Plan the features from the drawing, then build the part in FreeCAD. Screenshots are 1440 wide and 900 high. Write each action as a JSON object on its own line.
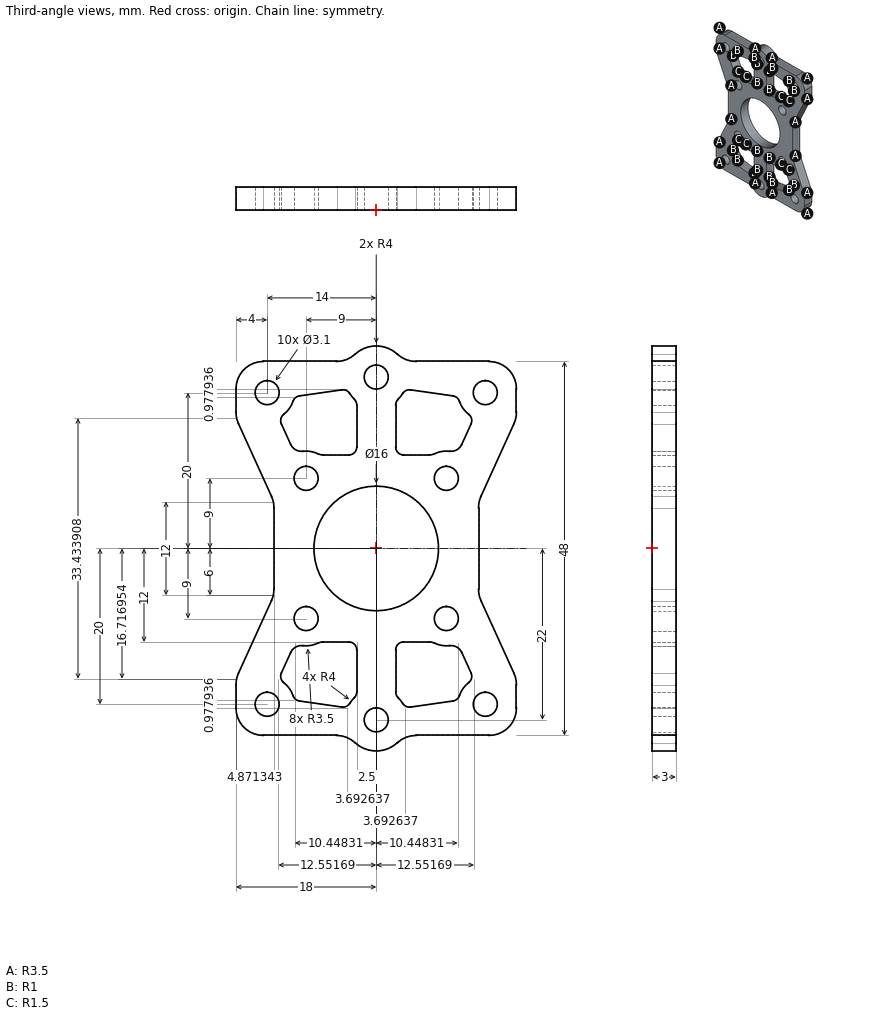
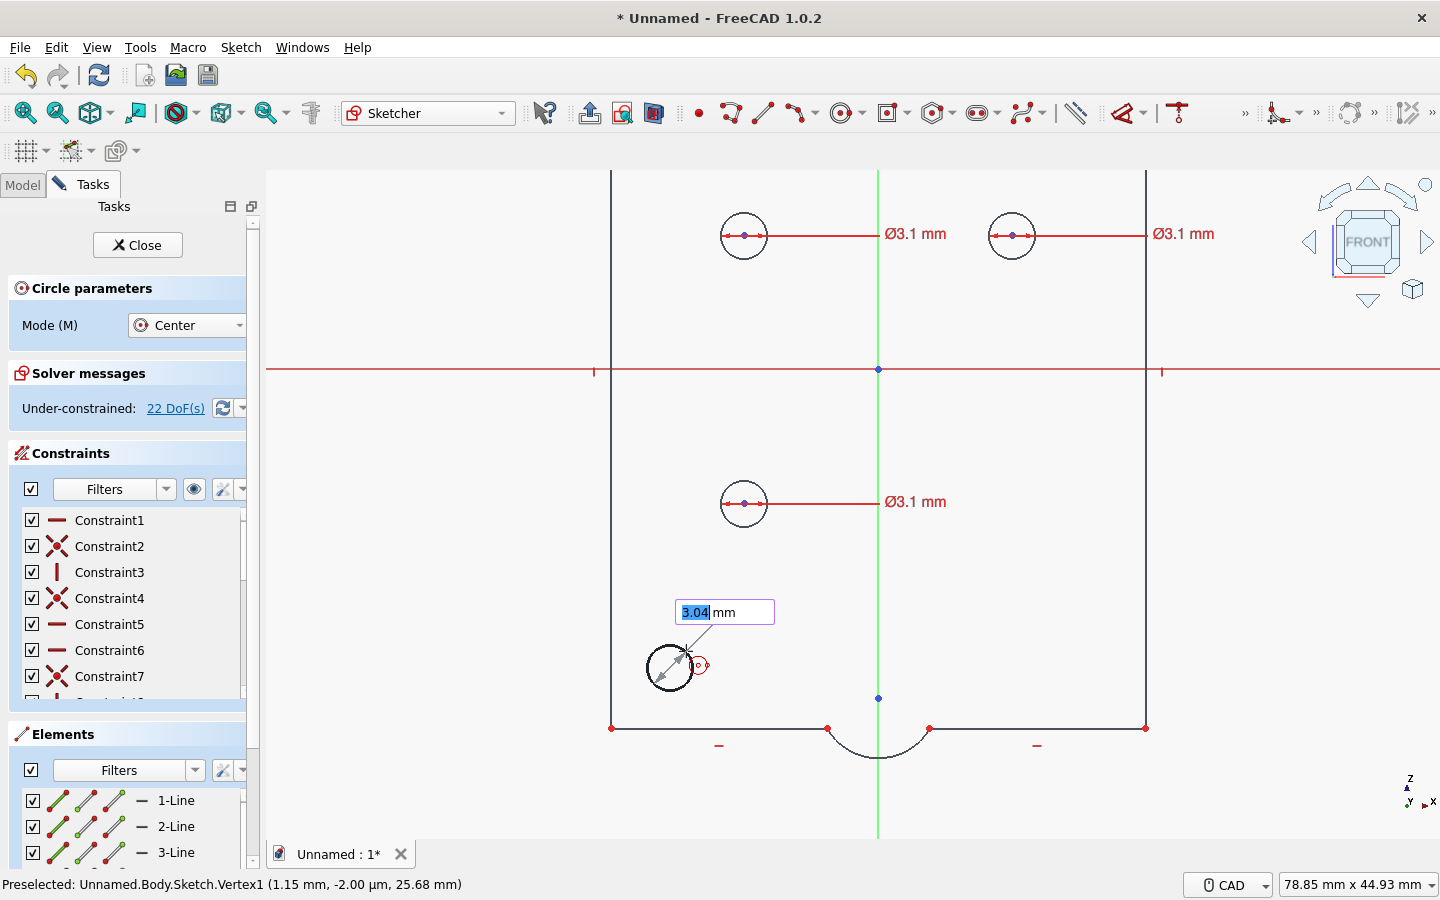
{"action": "type", "text": "3.1"}
{"action": "key", "text": "Return"}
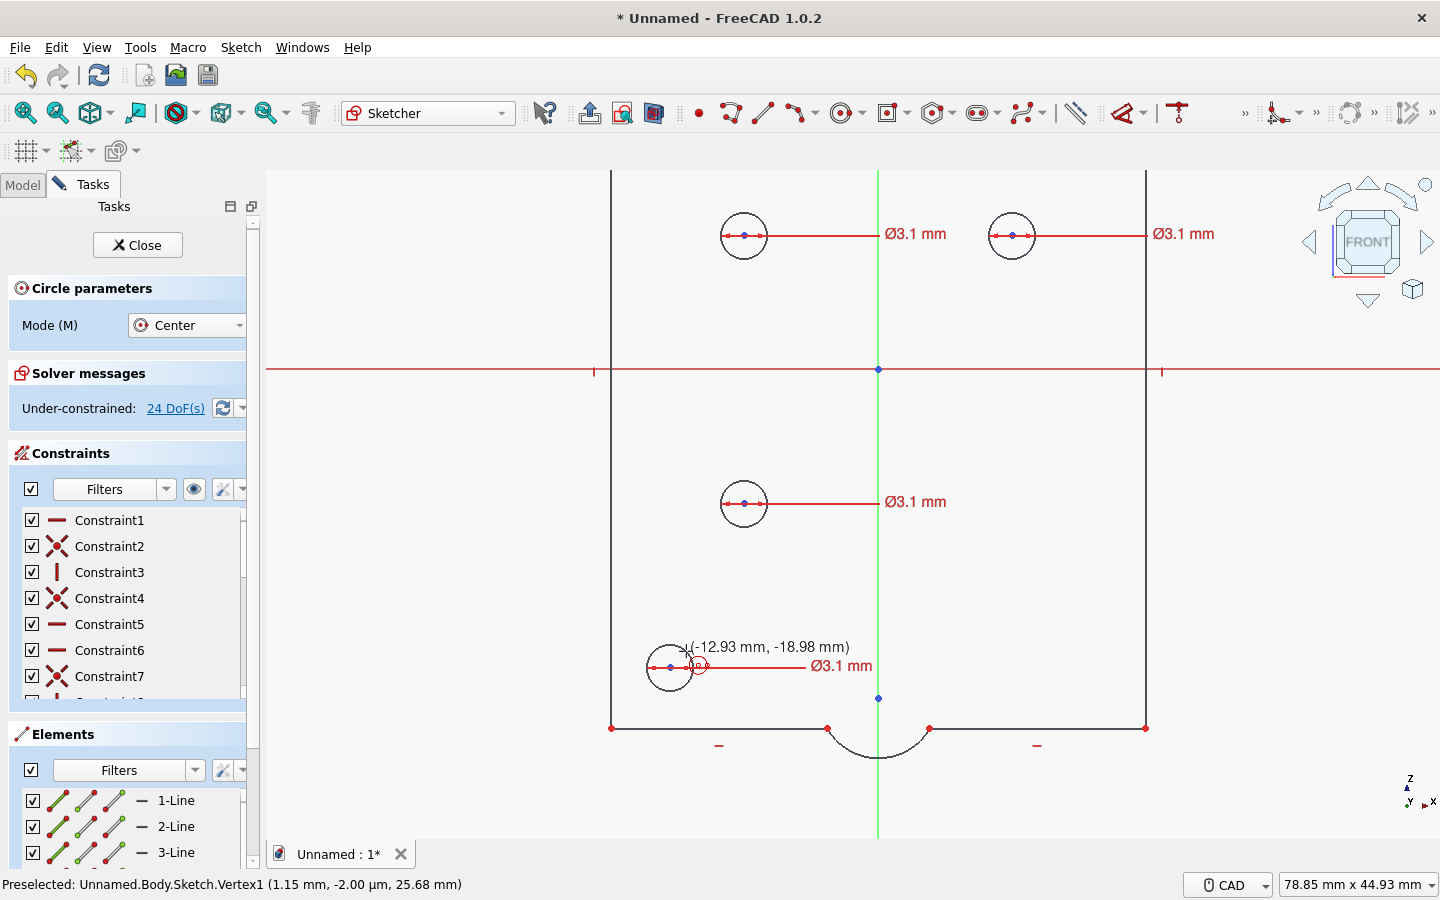
{"action": "left_click", "coordinate": [878, 369]}
{"action": "mouse_move", "coordinate": [963, 285]}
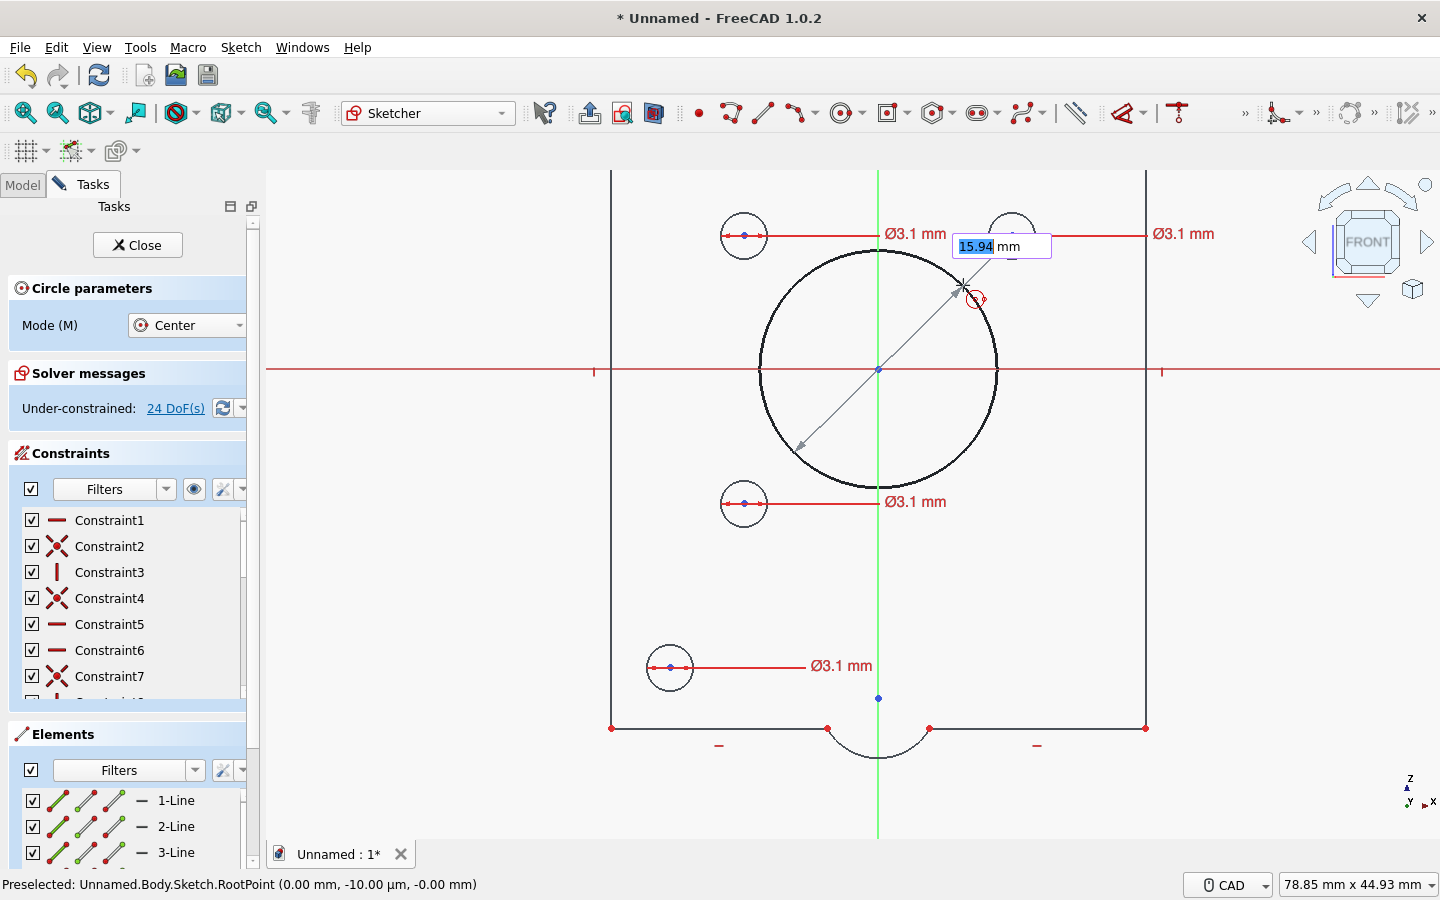
{"action": "type", "text": "16"}
{"action": "key", "text": "Return"}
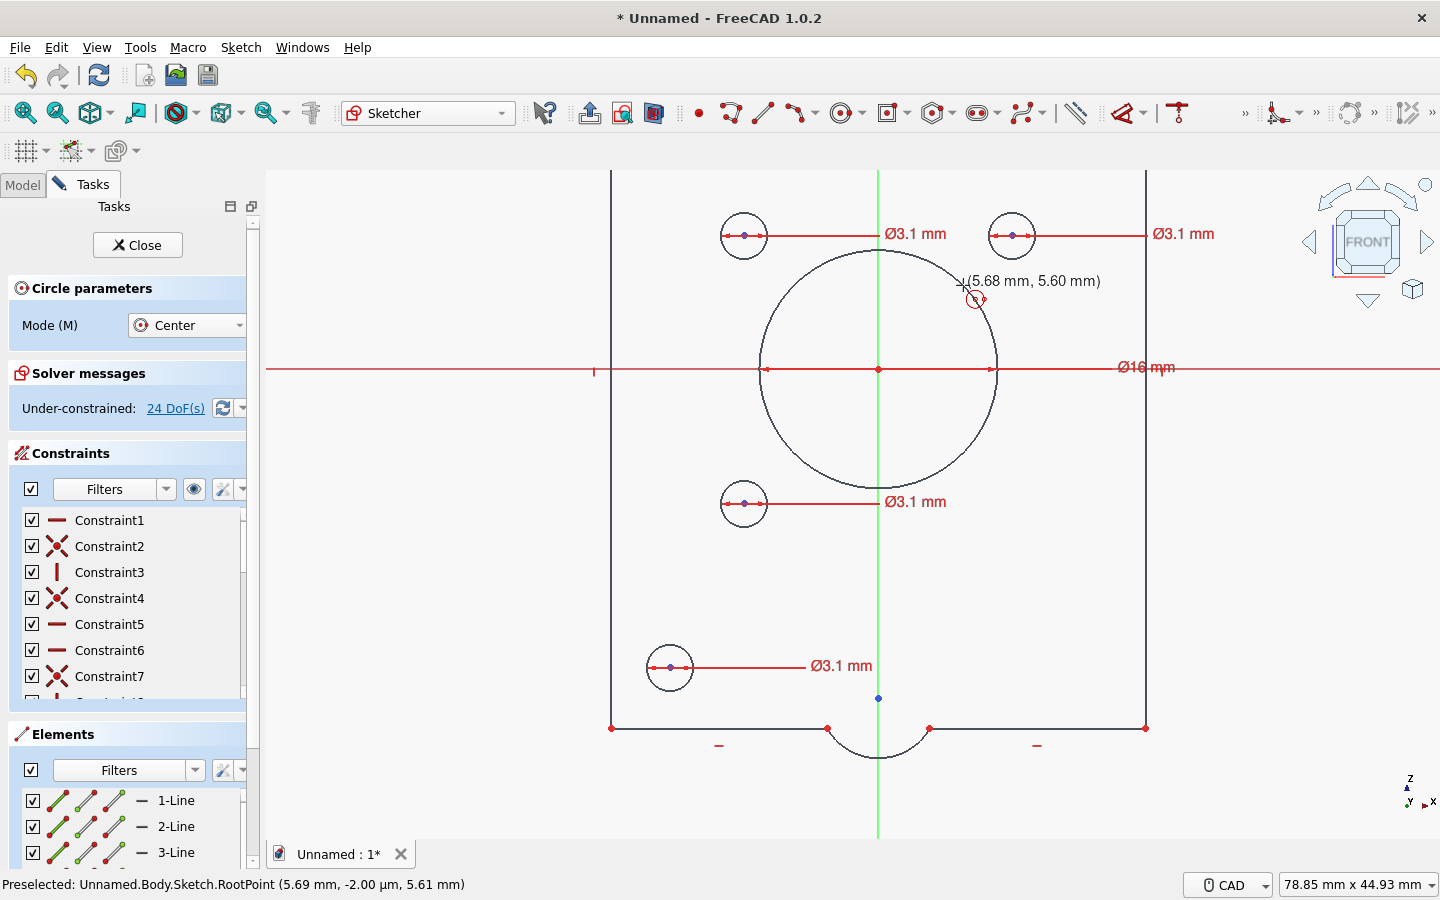
{"action": "left_click", "coordinate": [1012, 503]}
{"action": "mouse_move", "coordinate": [1029, 487]}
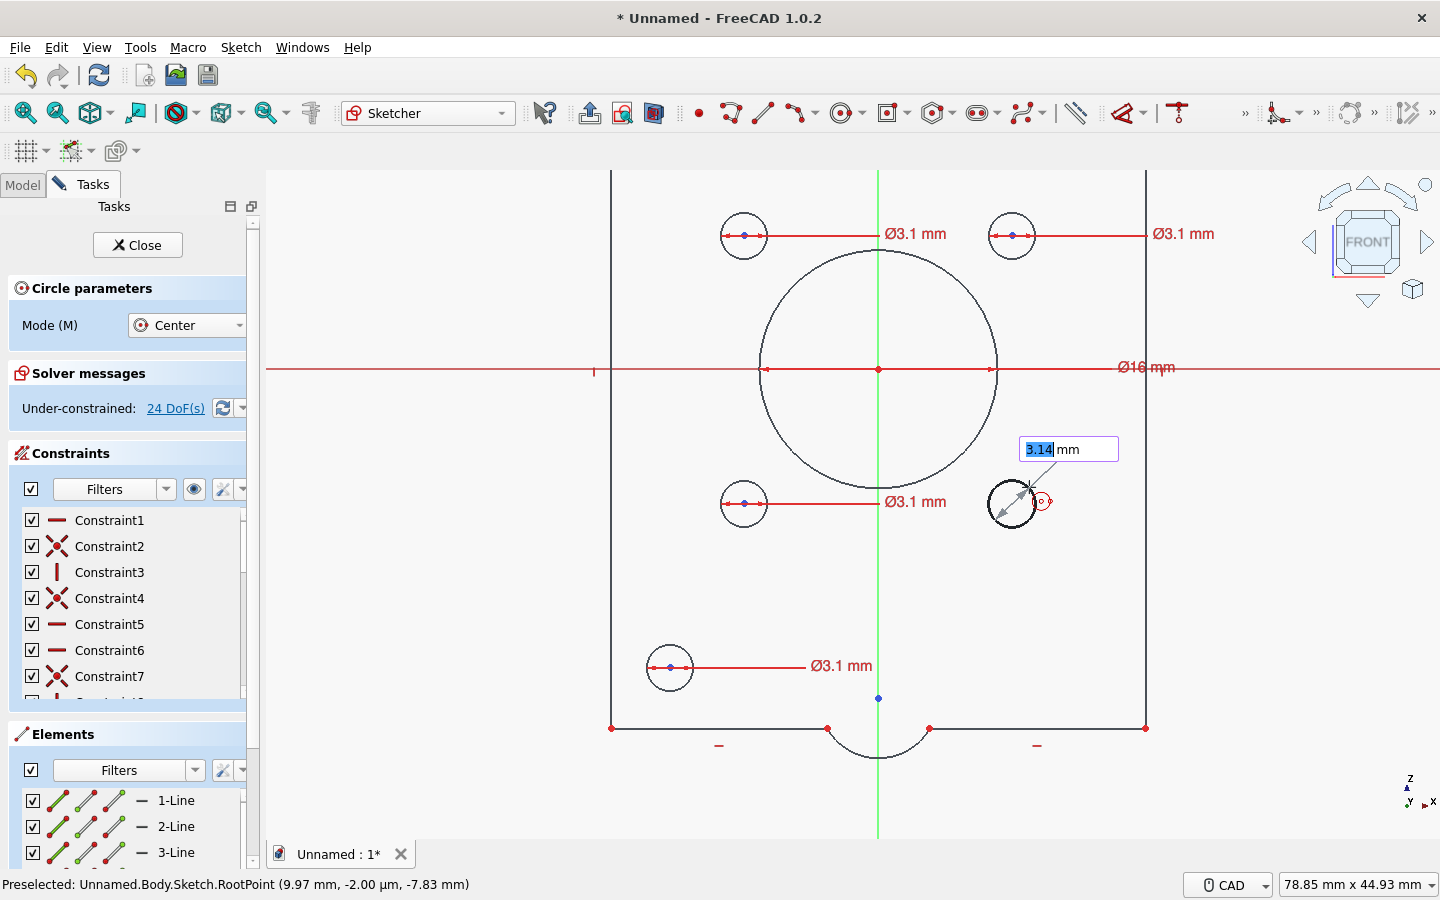
{"action": "type", "text": "3.1"}
{"action": "key", "text": "Return"}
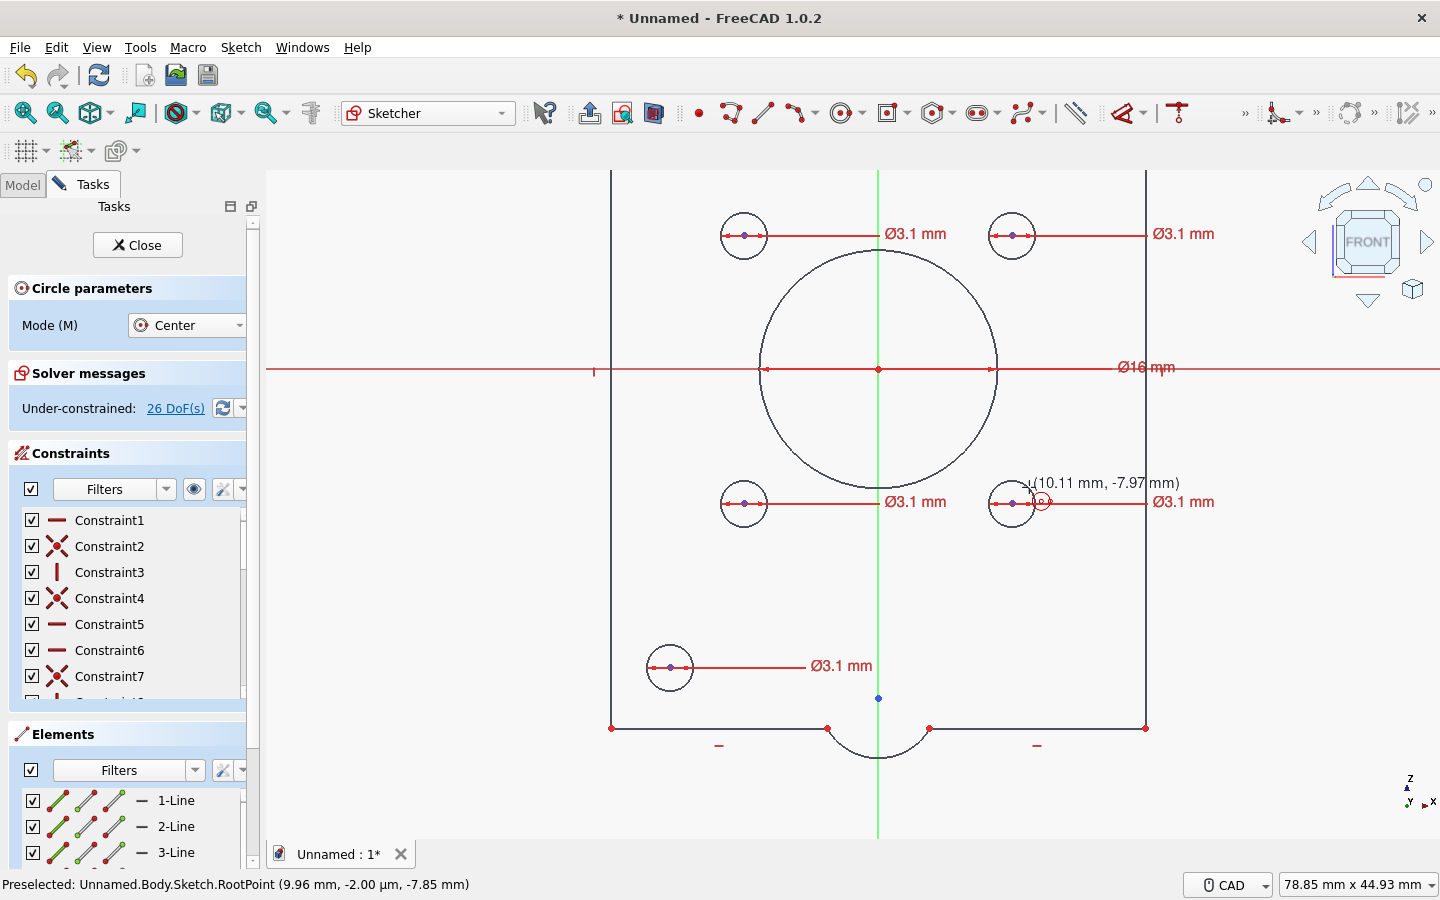
{"action": "left_click", "coordinate": [1087, 667]}
{"action": "mouse_move", "coordinate": [1103, 651]}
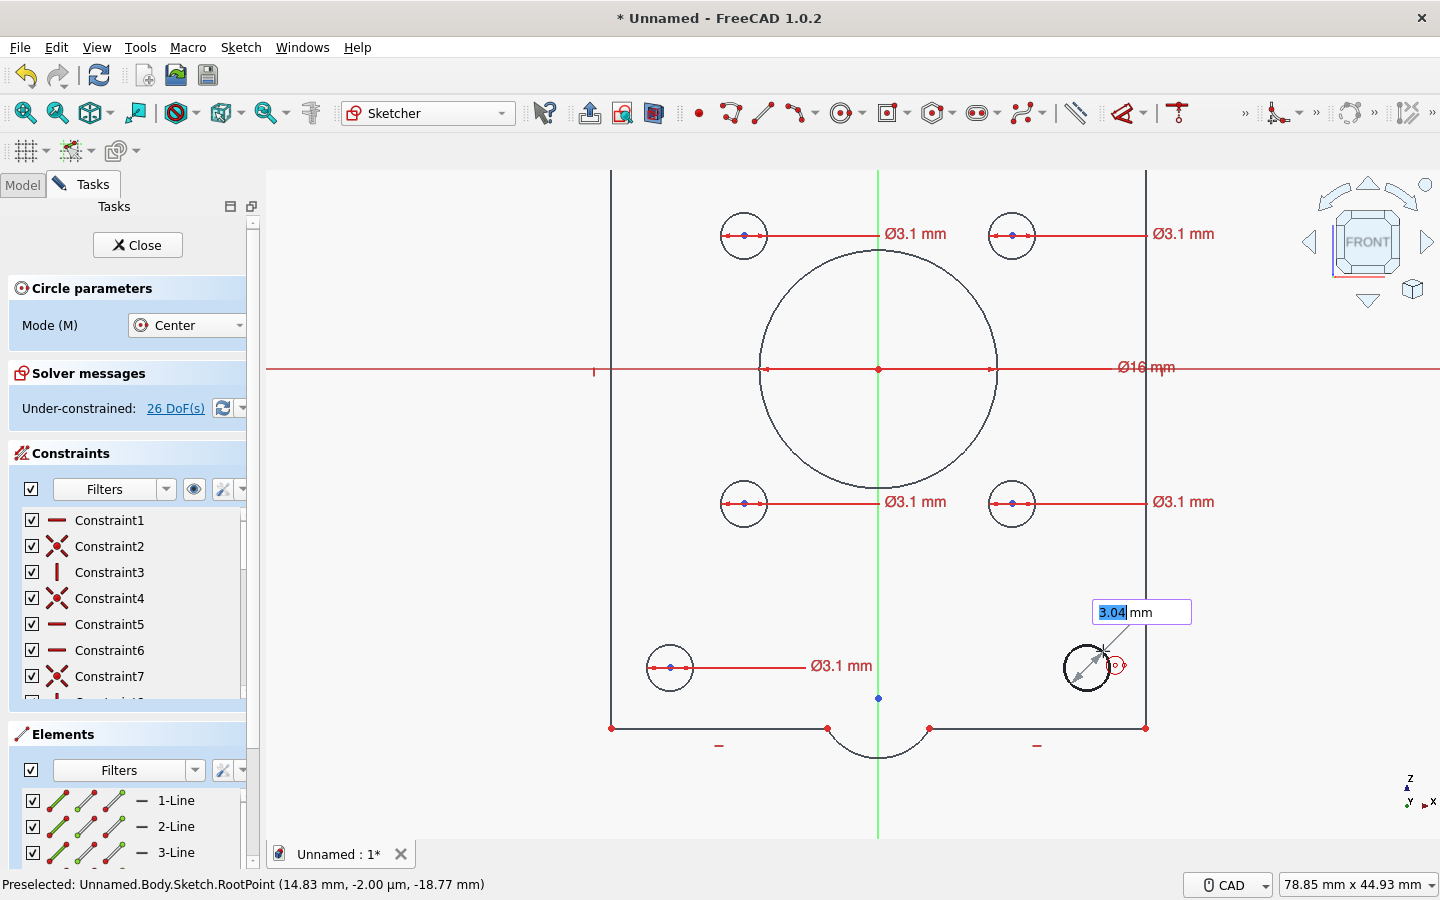
{"action": "type", "text": "3.1"}
{"action": "key", "text": "Return"}